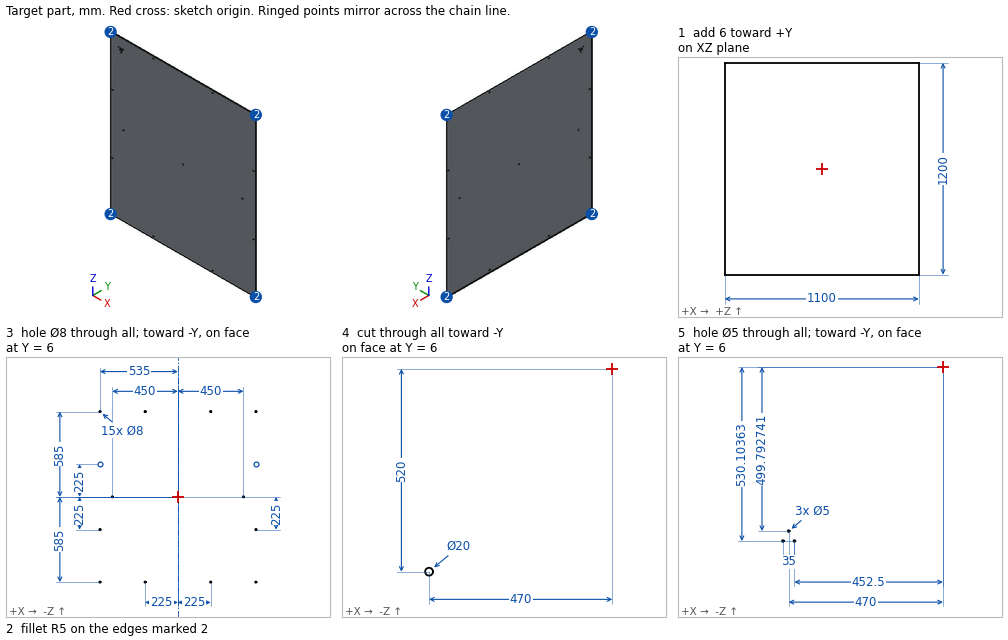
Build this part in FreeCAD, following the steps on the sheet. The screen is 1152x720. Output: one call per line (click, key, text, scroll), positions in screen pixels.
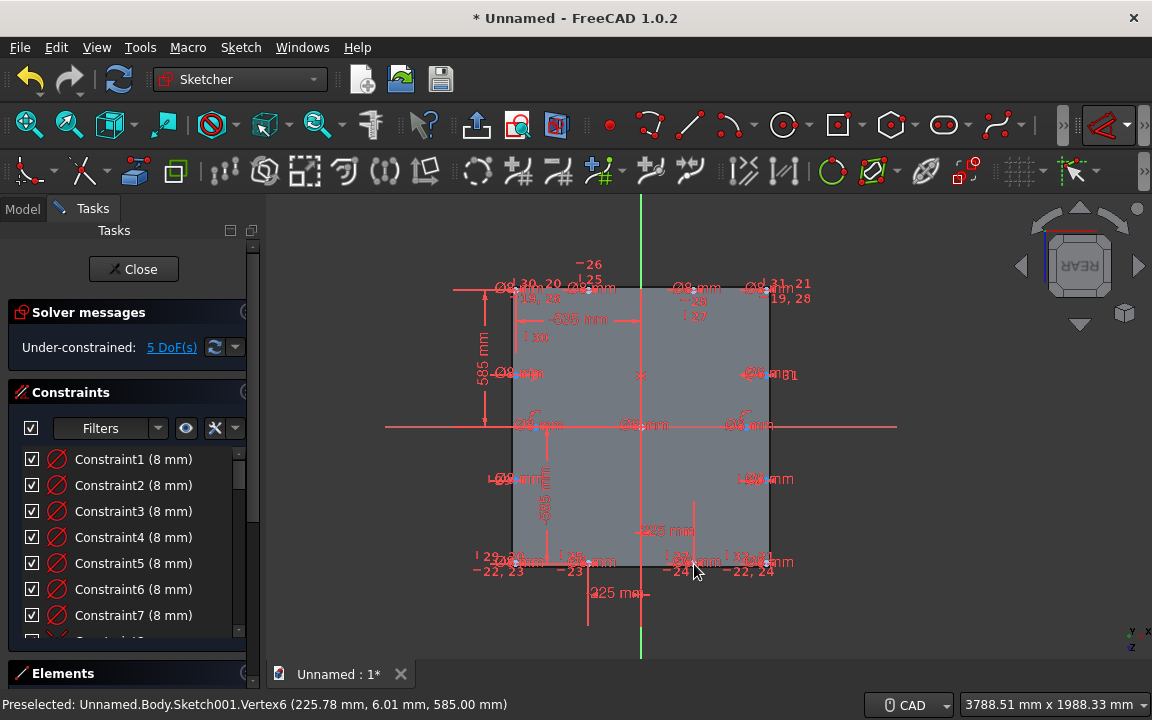
click(516, 481)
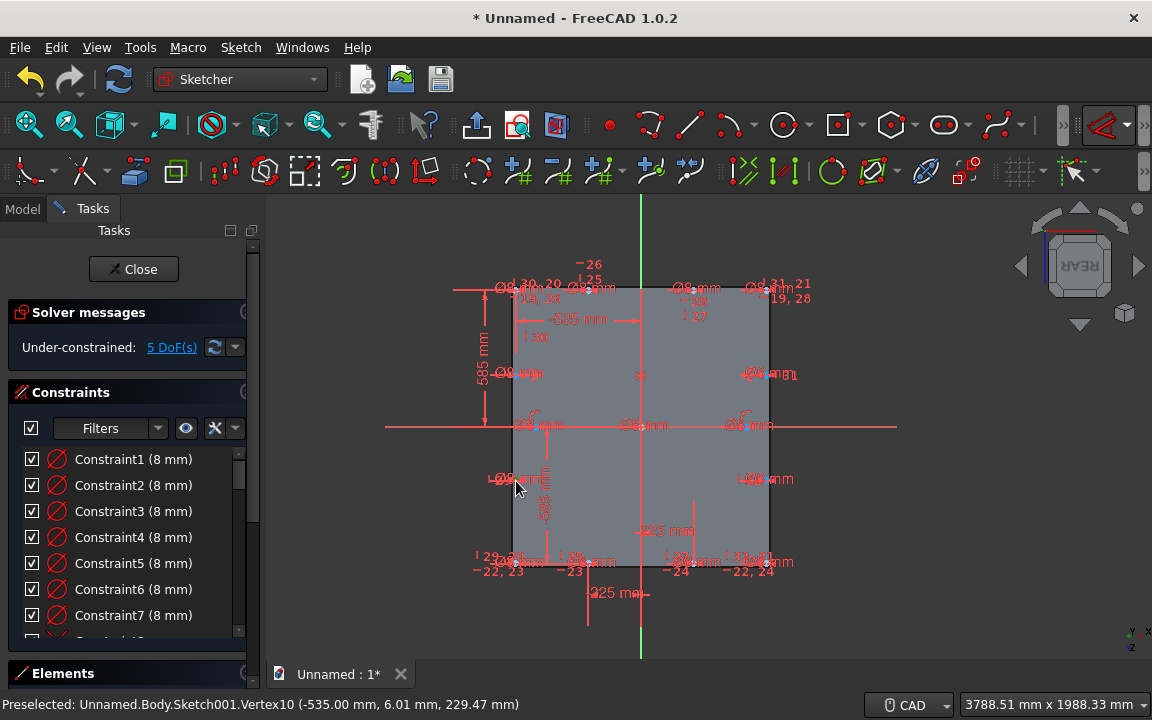
key(i)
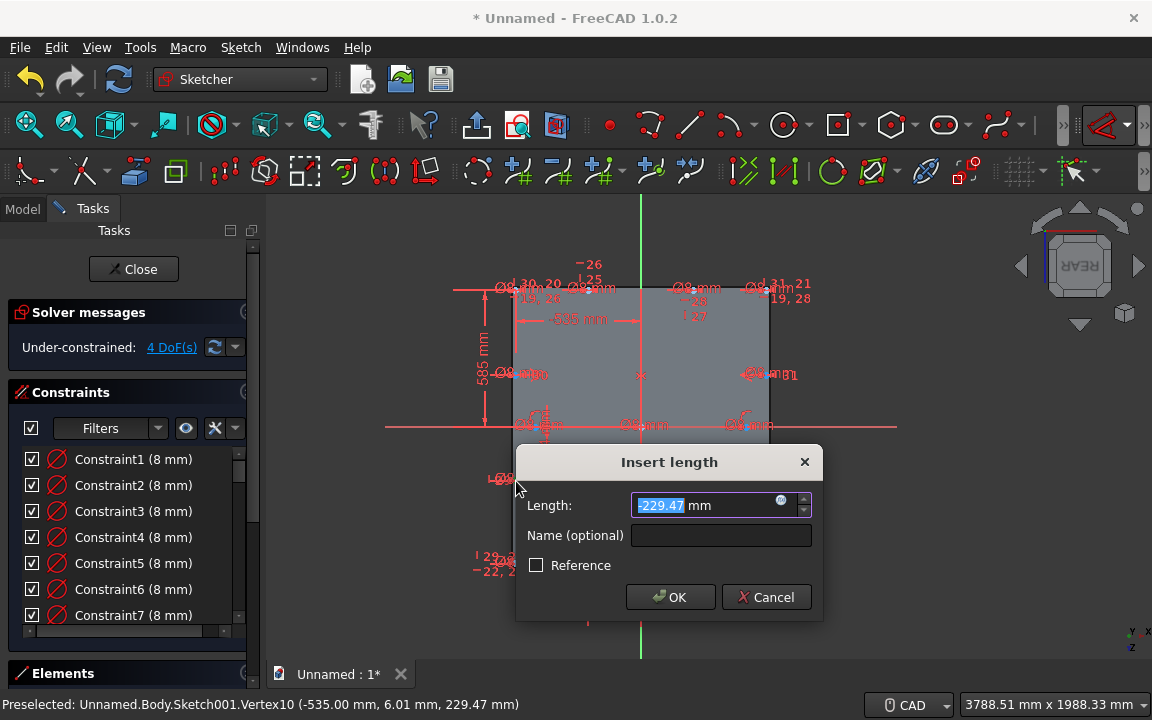
text(-225)
key(Return)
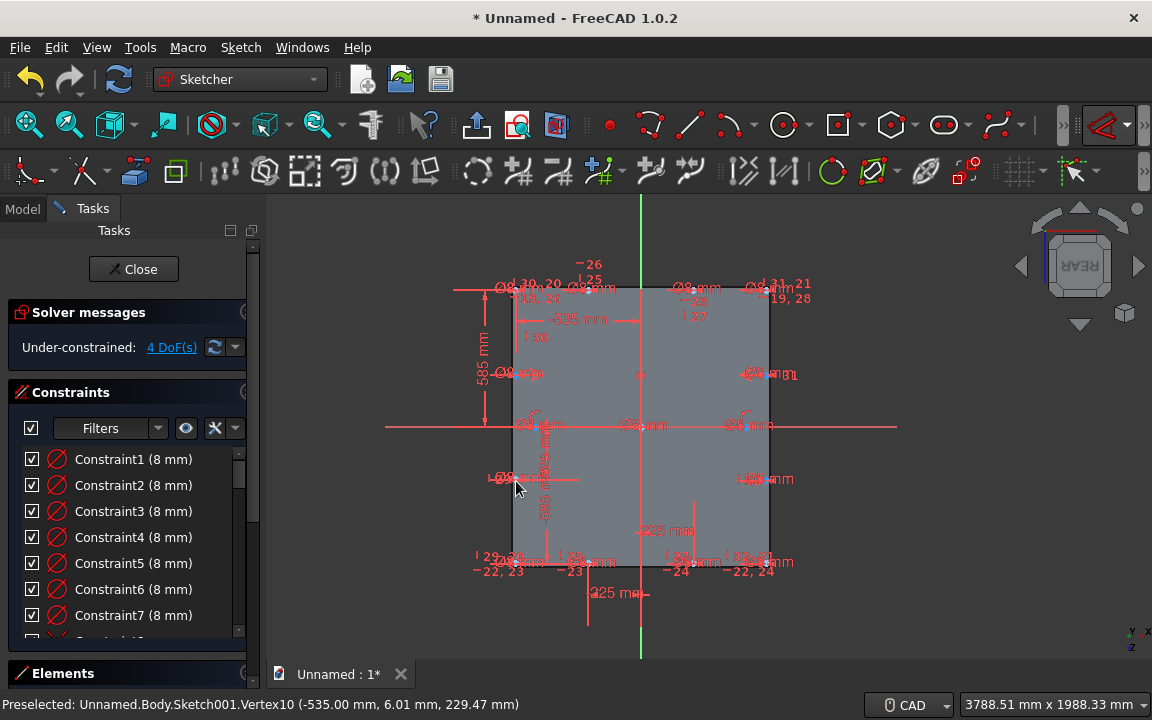
click(516, 375)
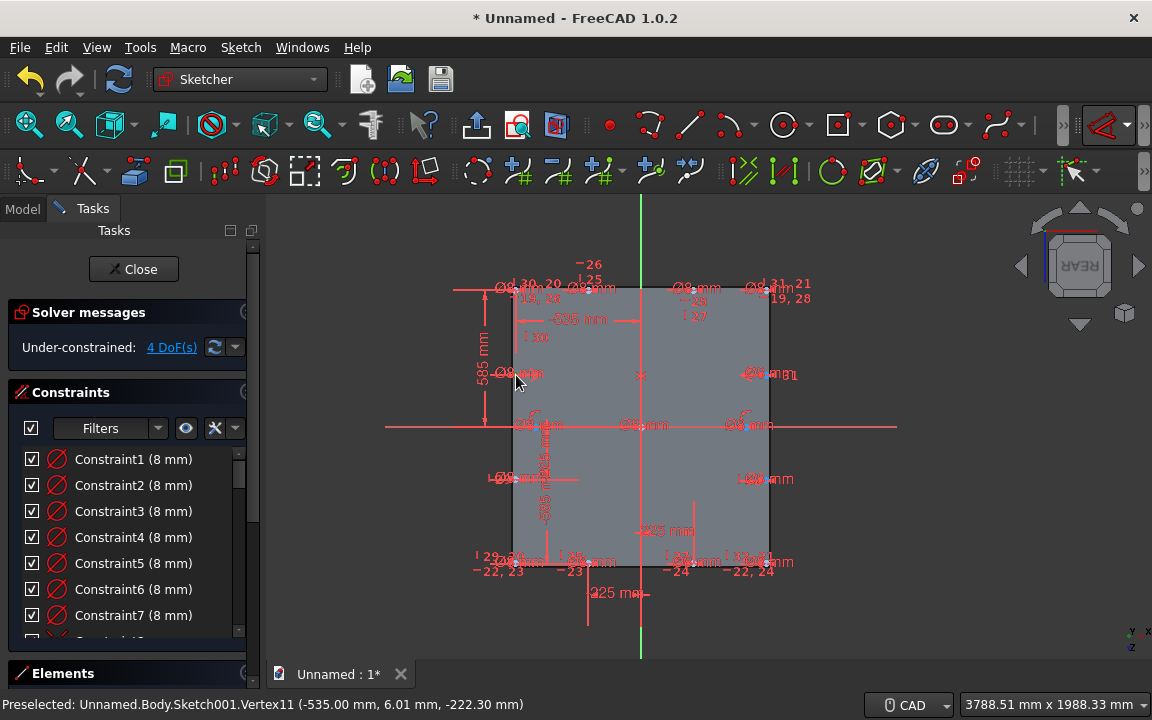
click(1130, 126)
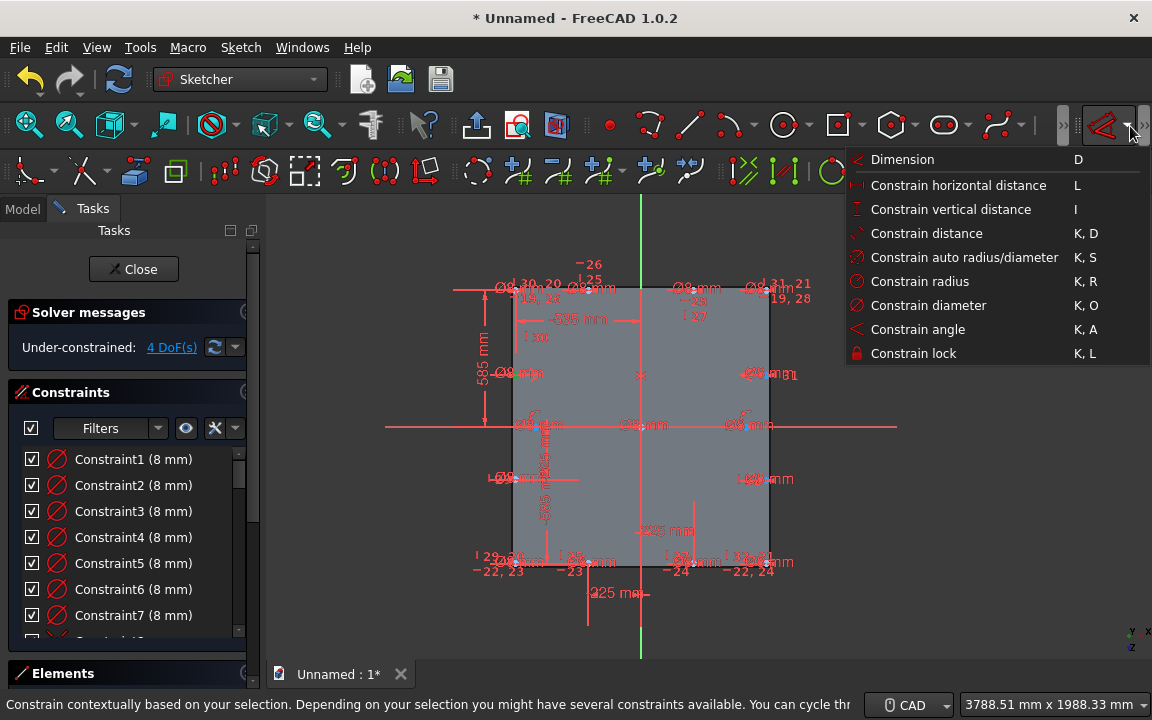
click(998, 209)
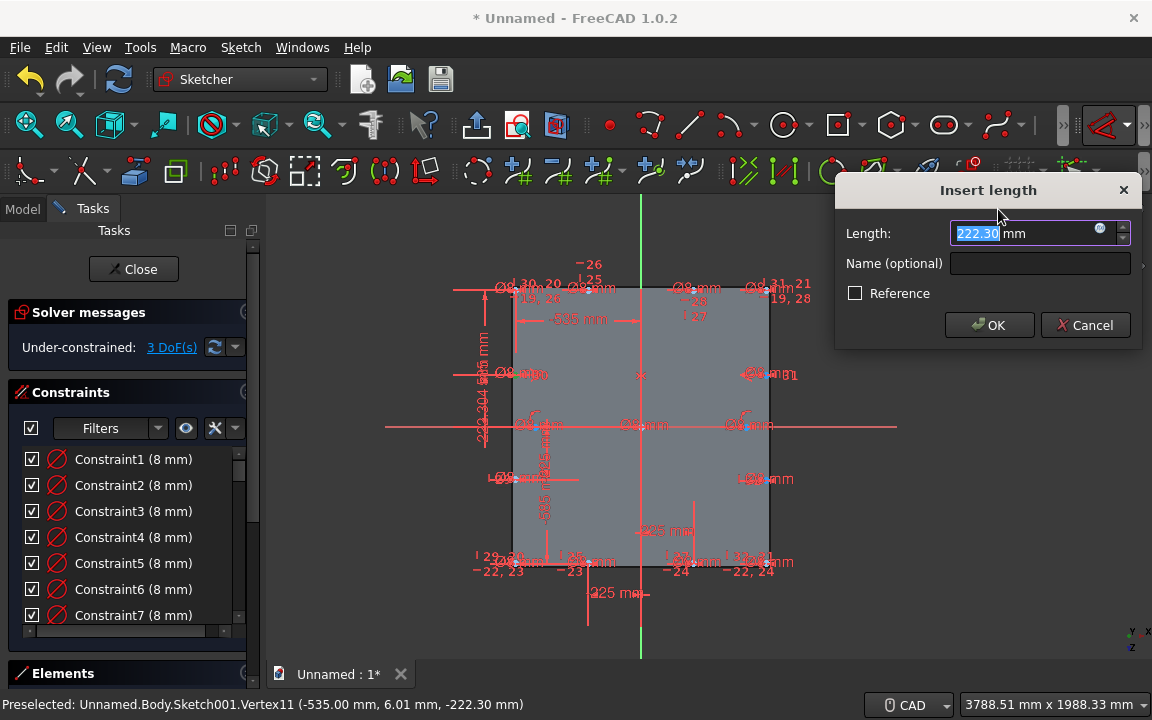
text(225)
key(Return)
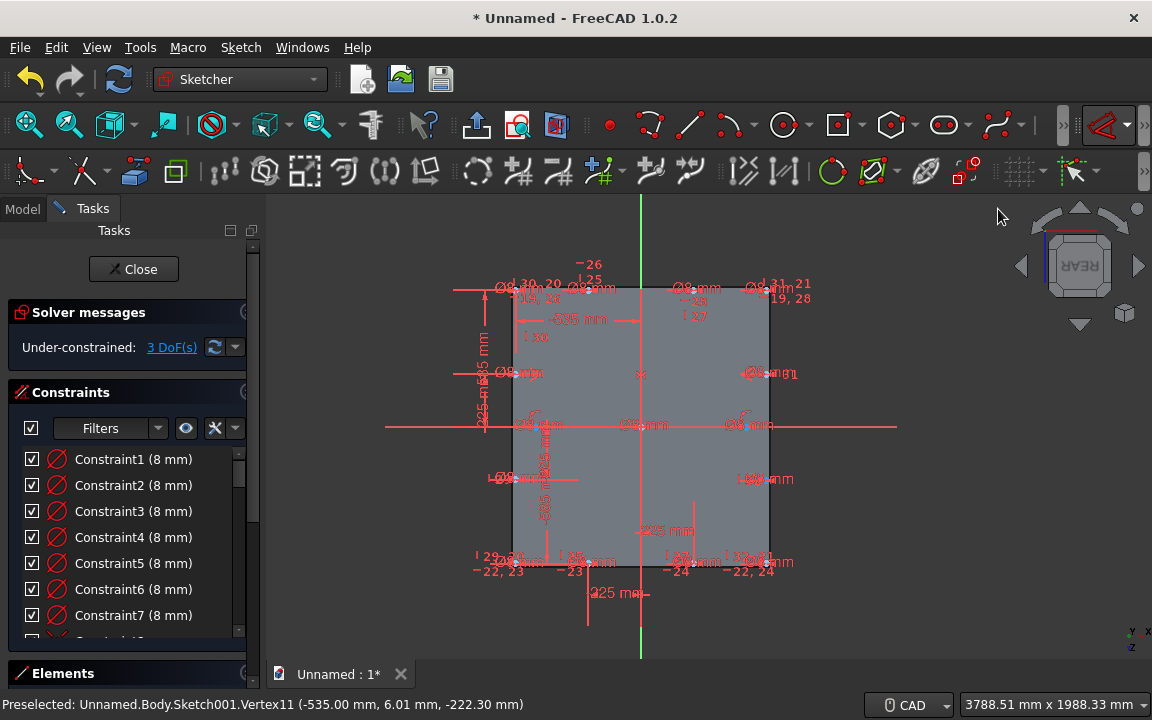
click(766, 481)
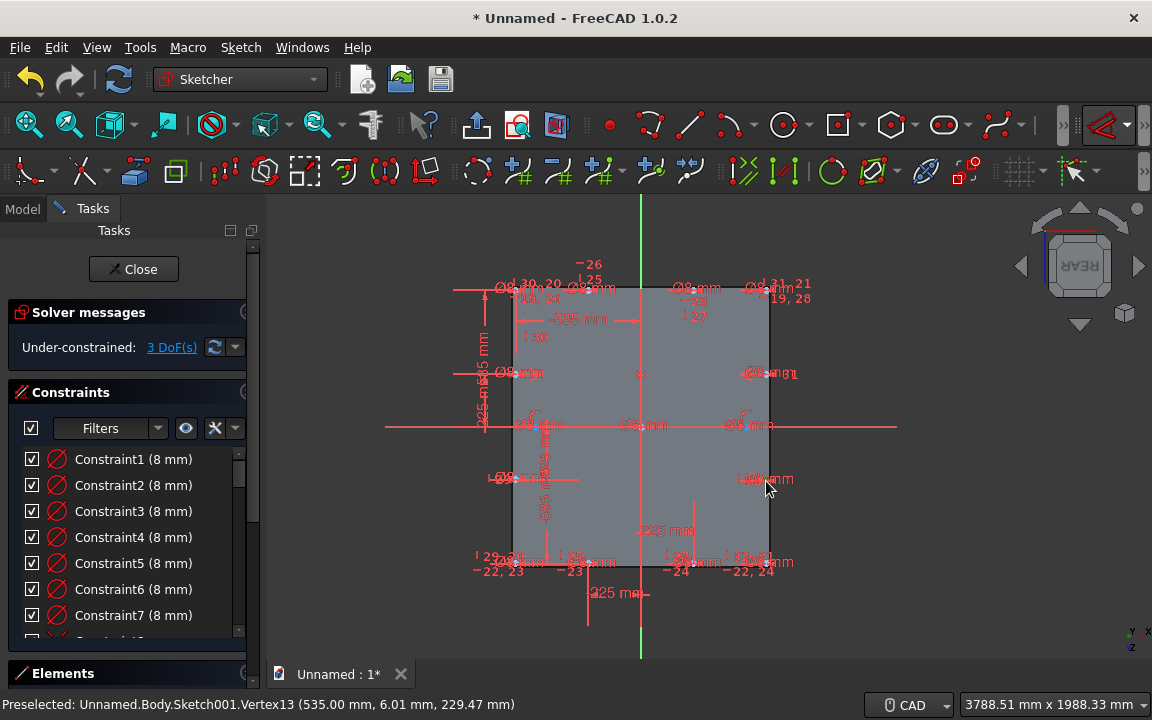
key(i)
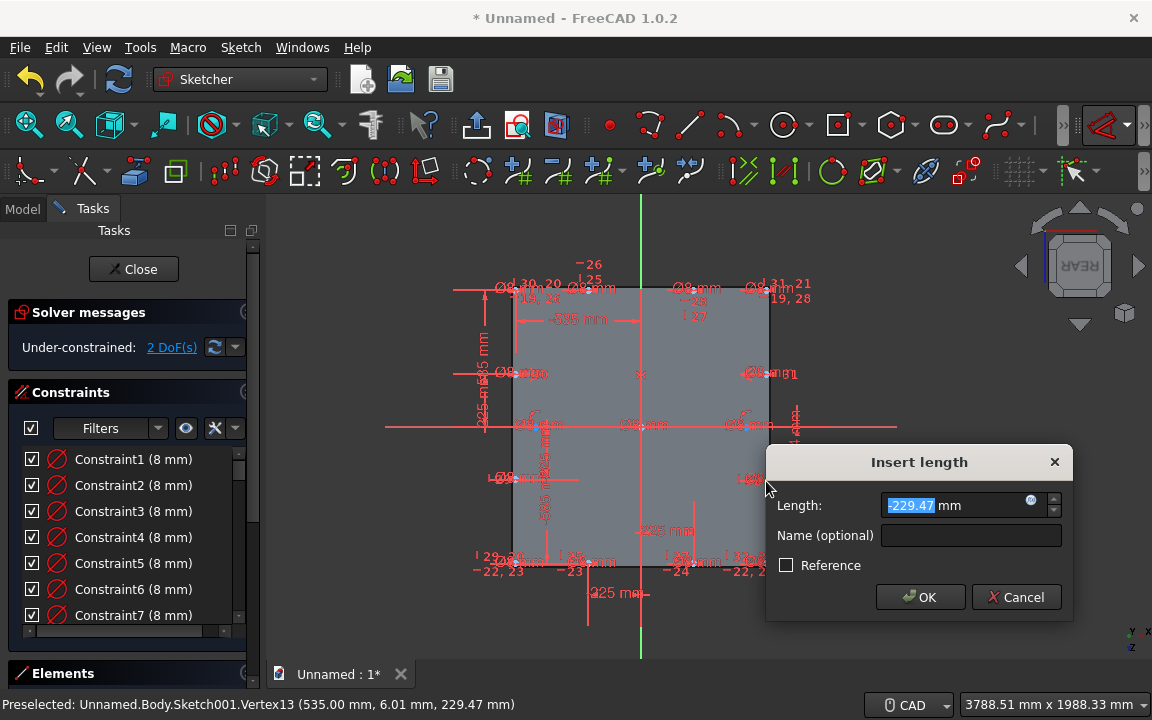
text(-225)
key(Return)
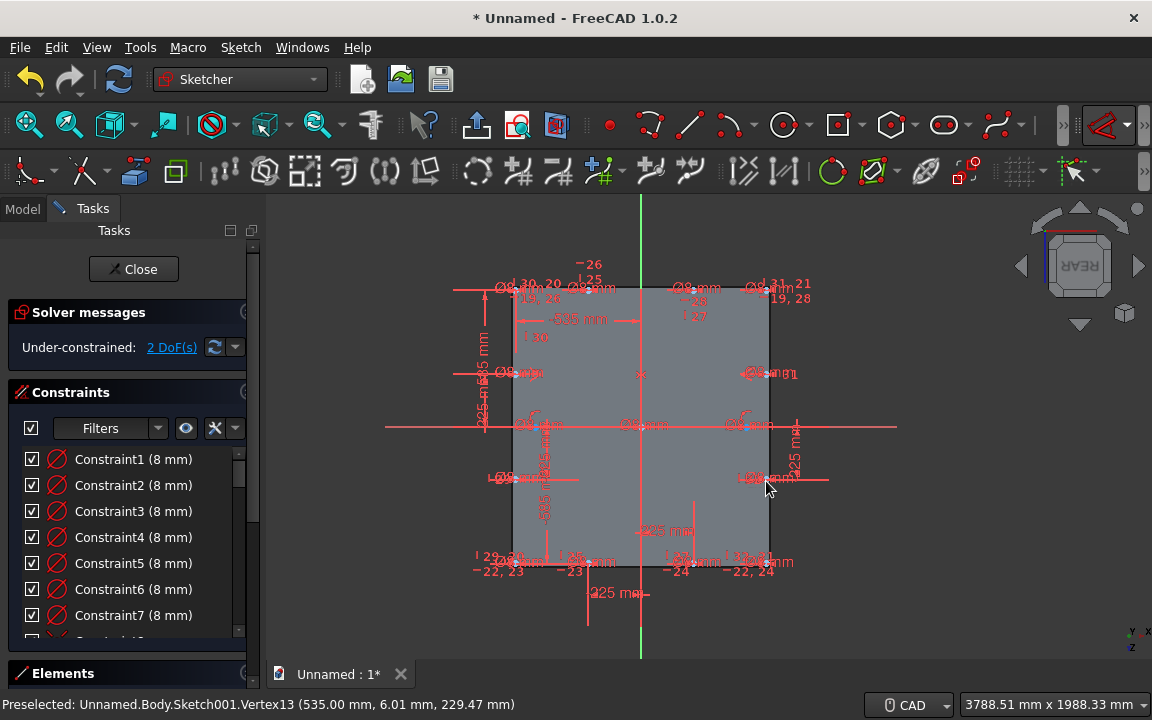
click(536, 427)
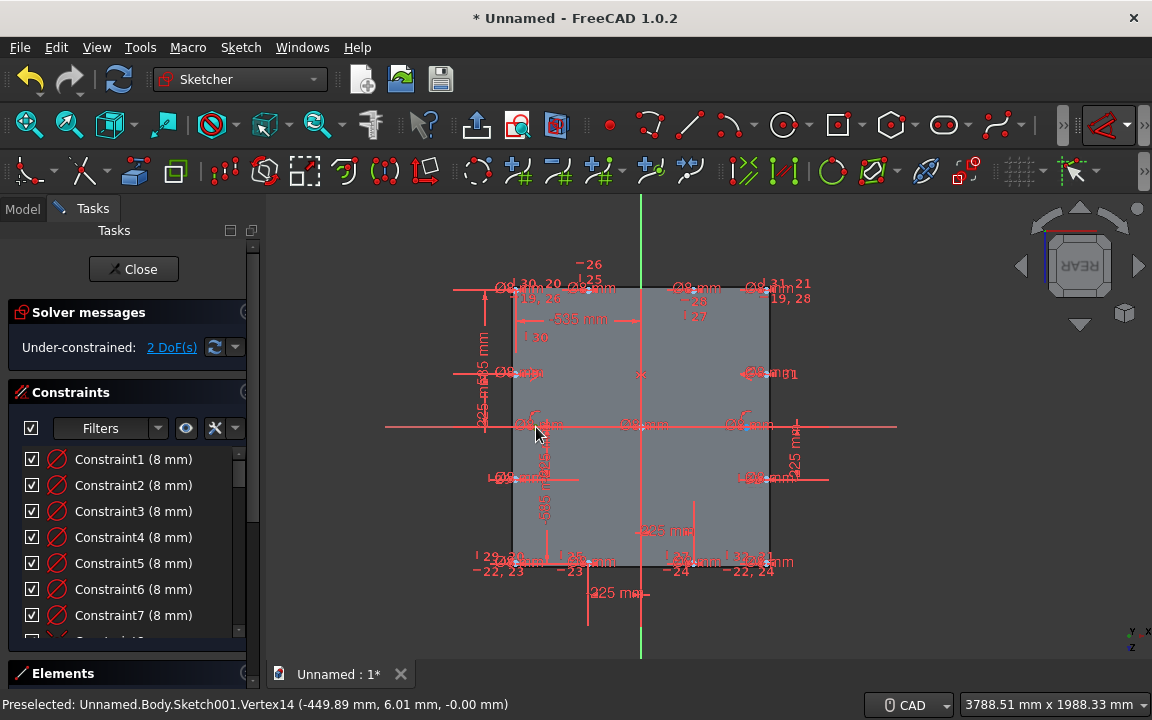
key(l)